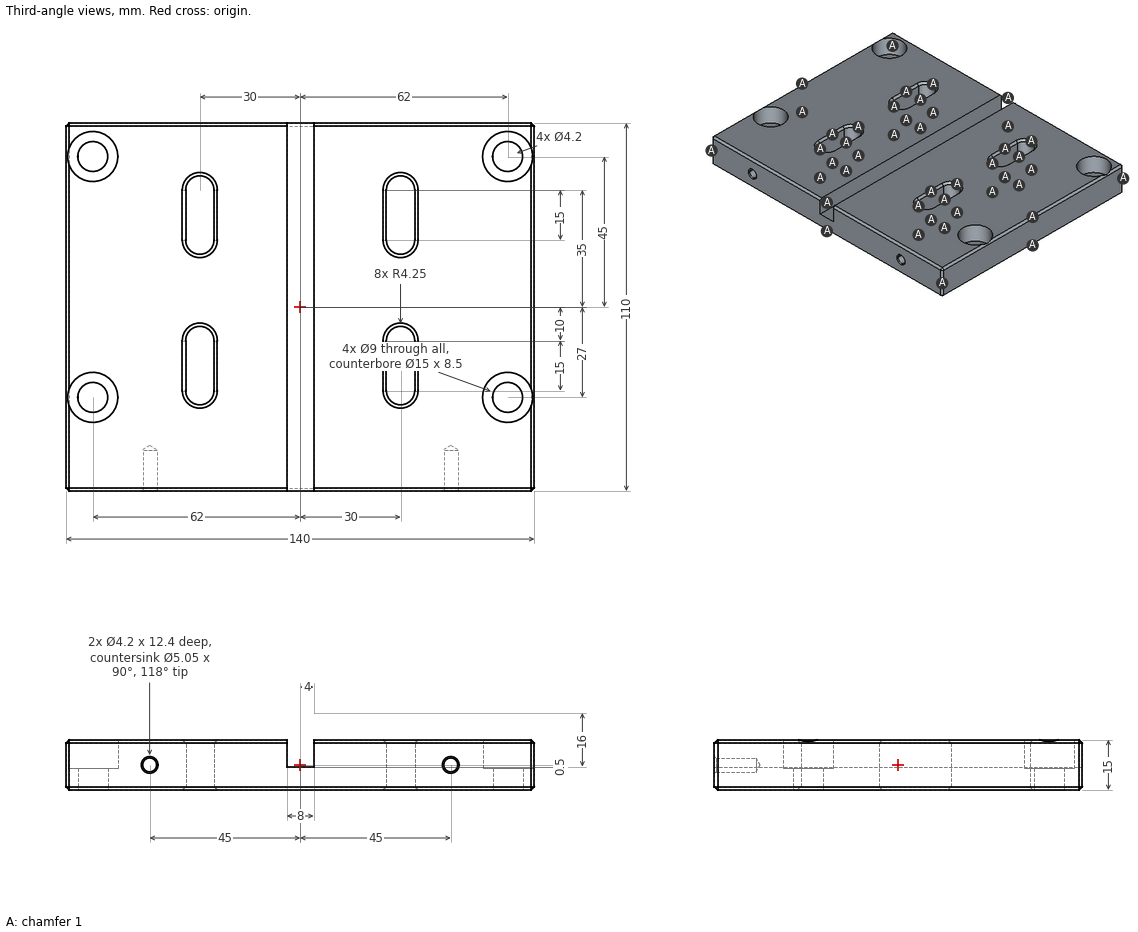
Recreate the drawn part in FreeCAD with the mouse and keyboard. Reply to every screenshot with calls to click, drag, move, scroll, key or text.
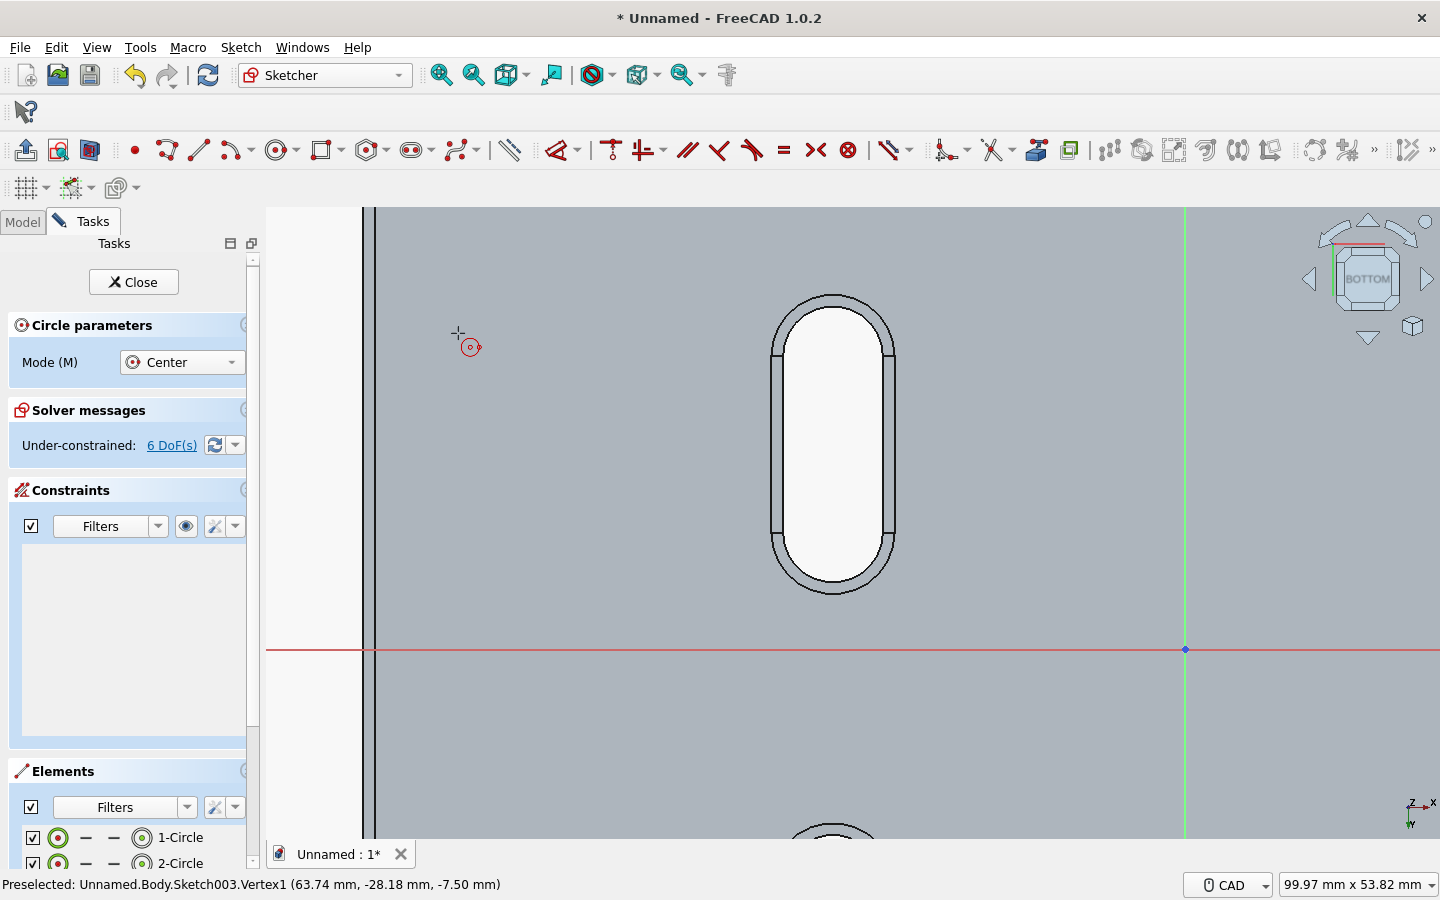
click(457, 333)
click(475, 315)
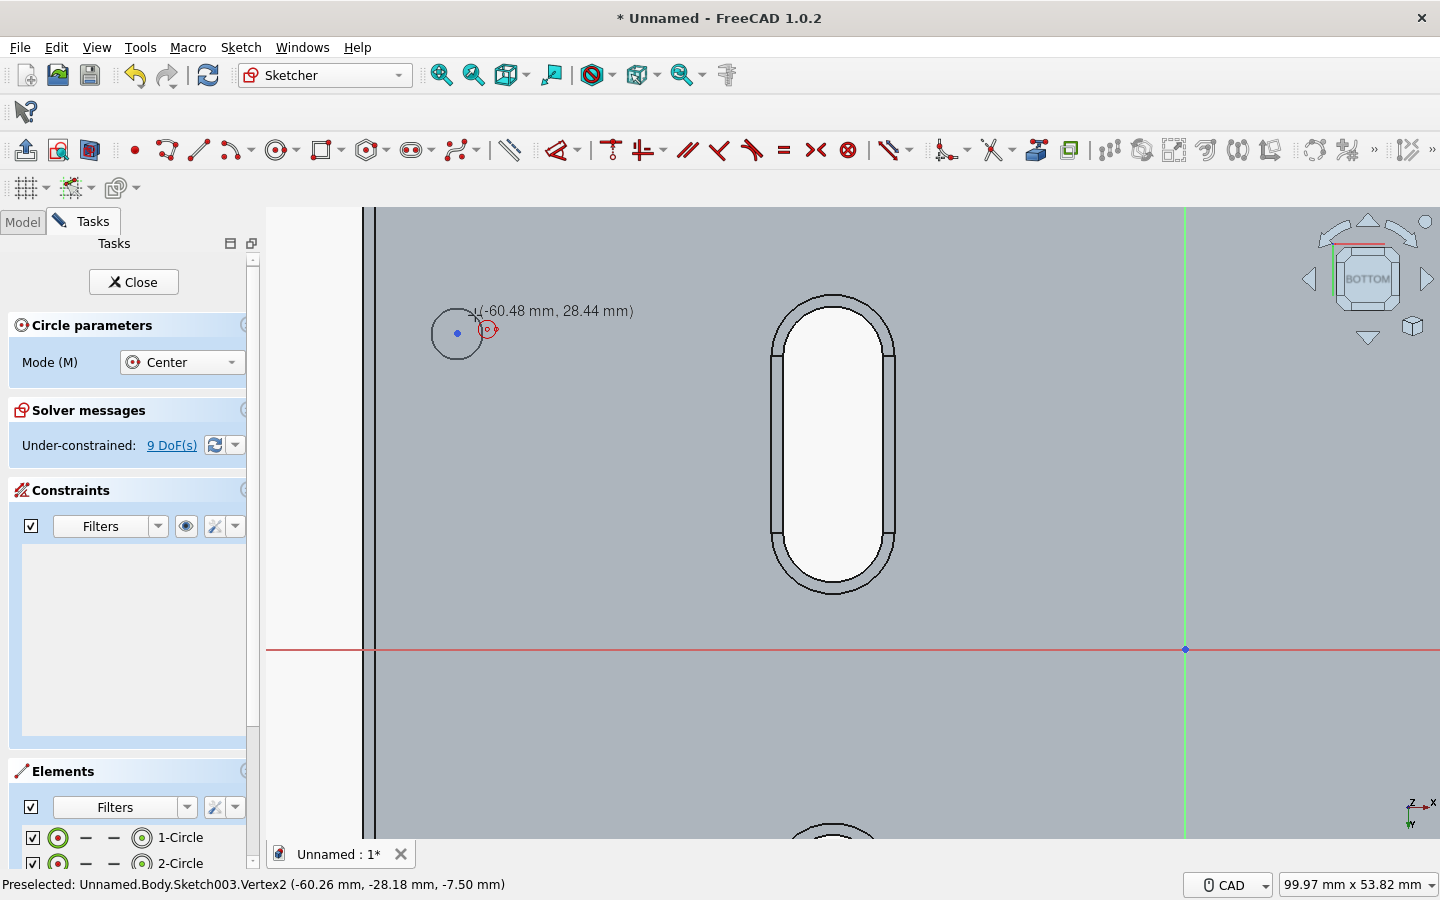
scroll(457, 333, down, 4)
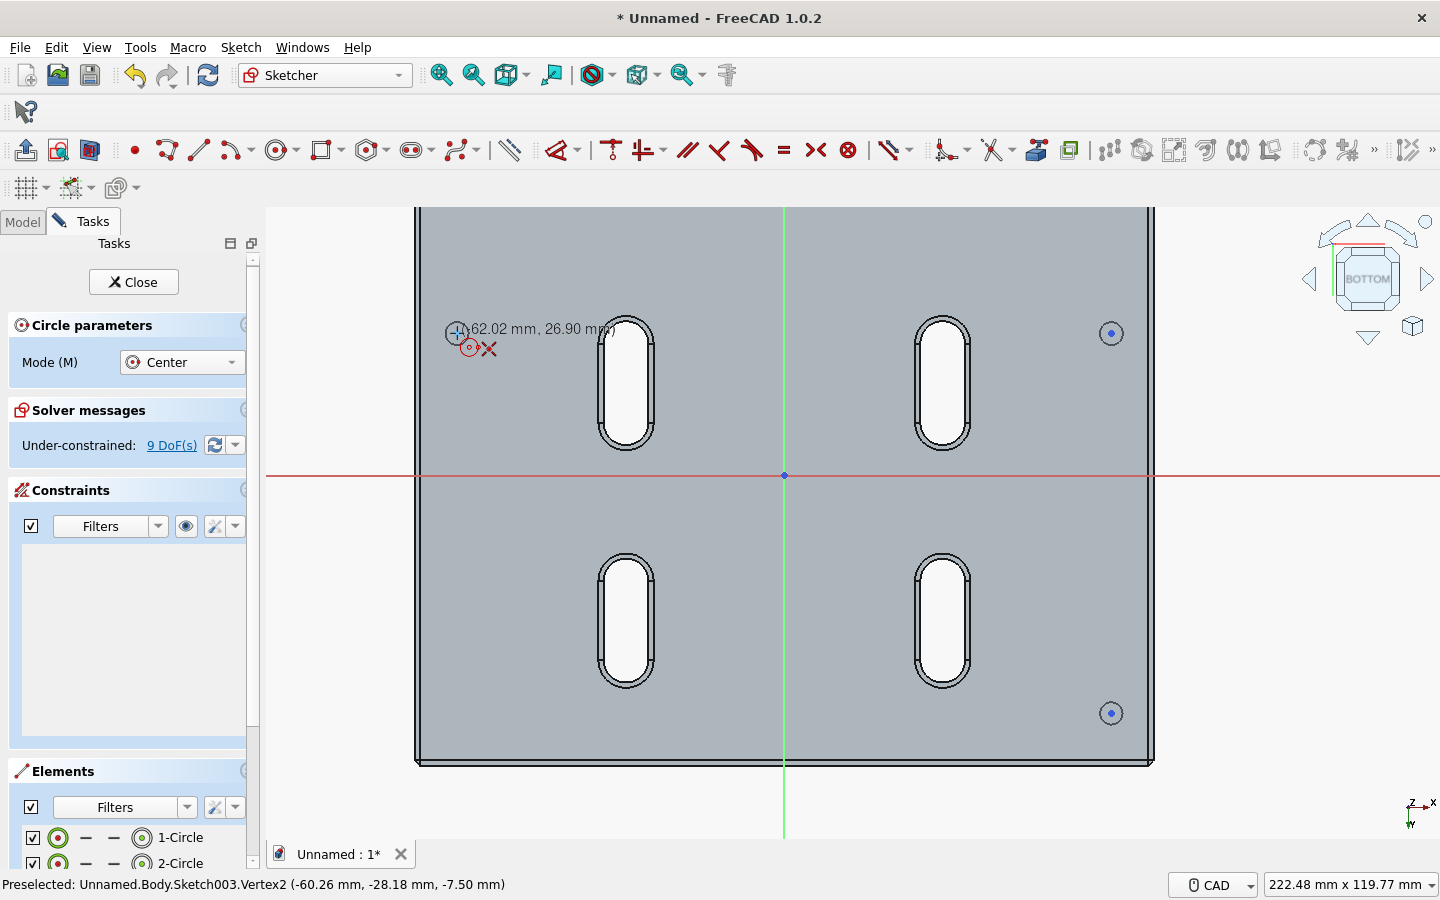
scroll(457, 713, up, 4)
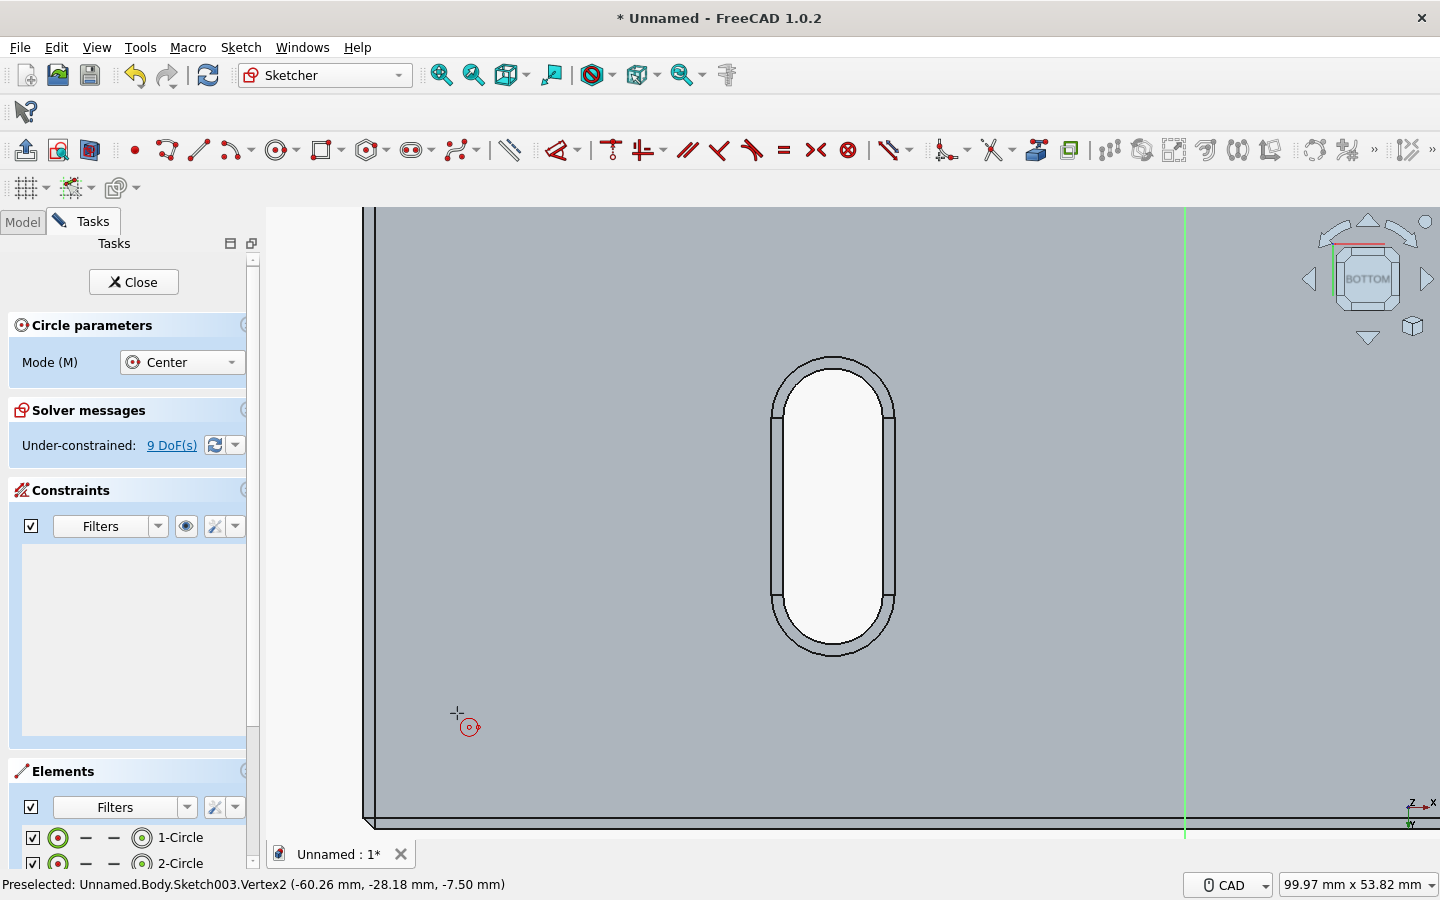
click(457, 712)
click(475, 695)
key(Escape)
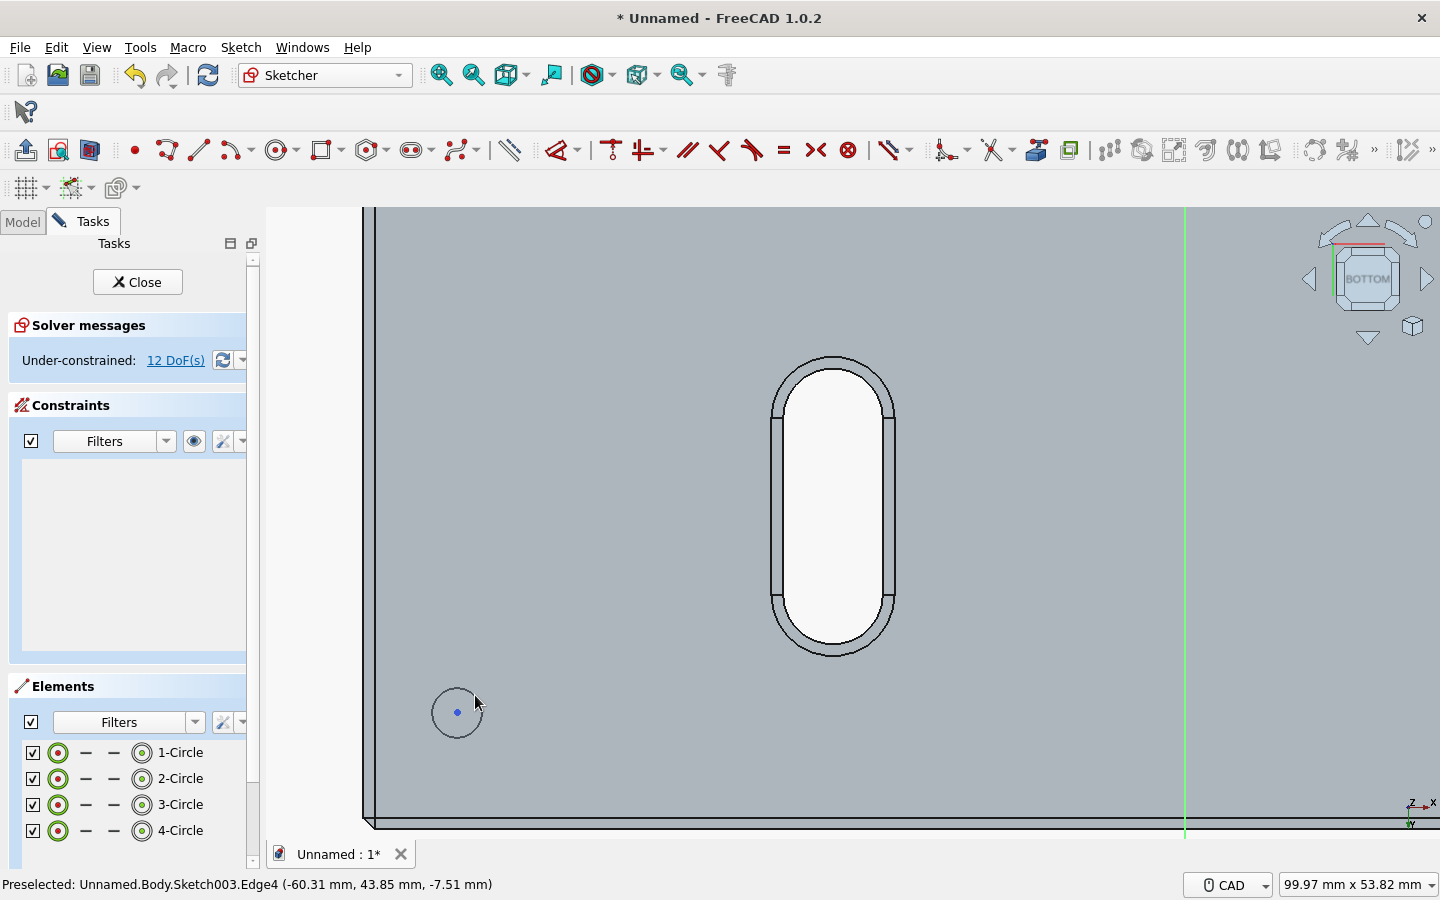
scroll(457, 714, down, 4)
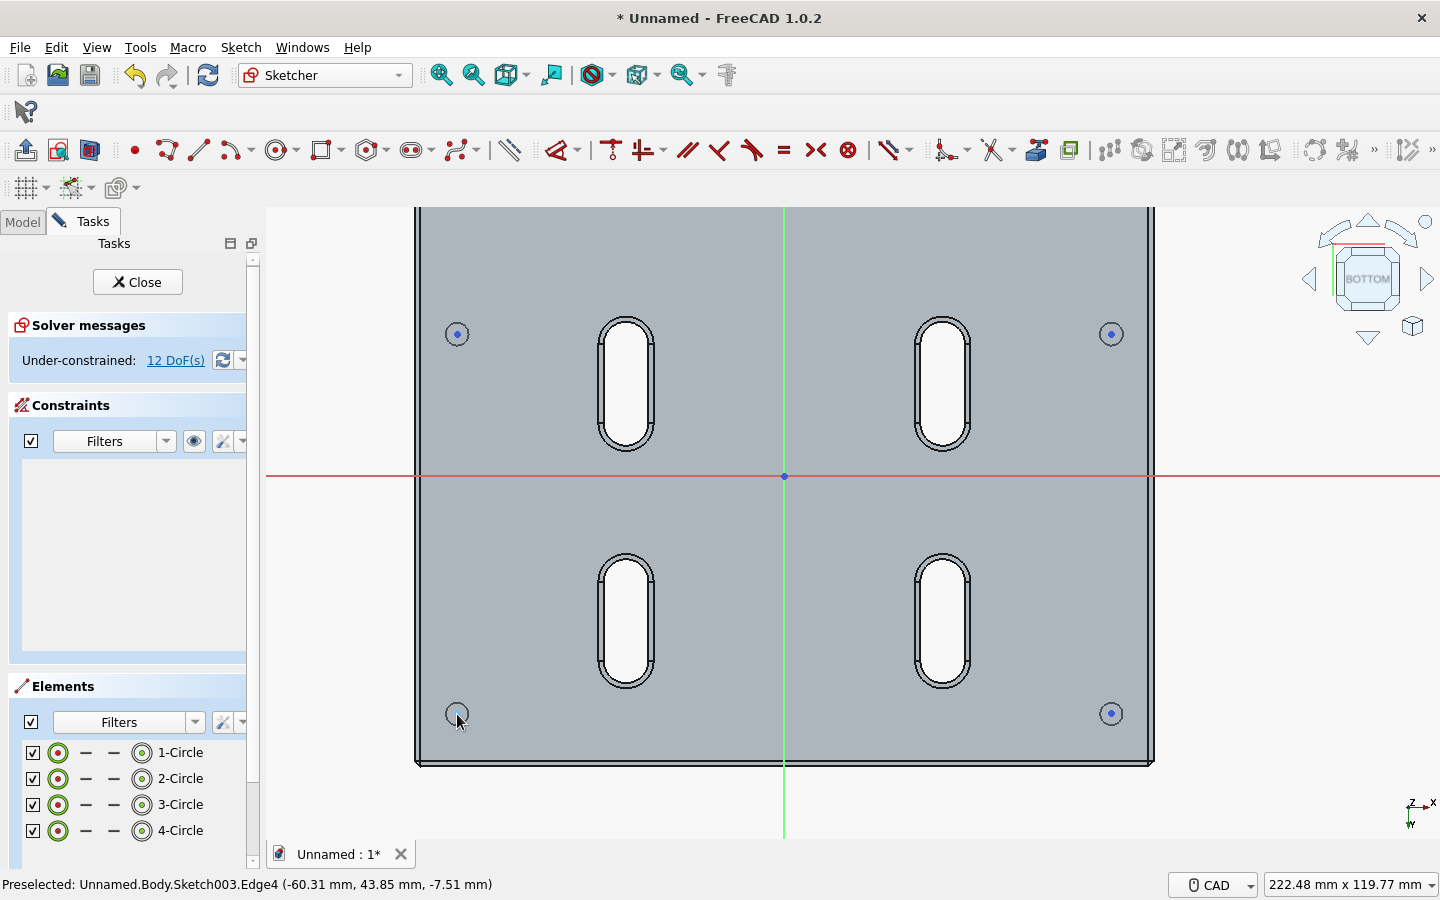
scroll(1119, 706, up, 2)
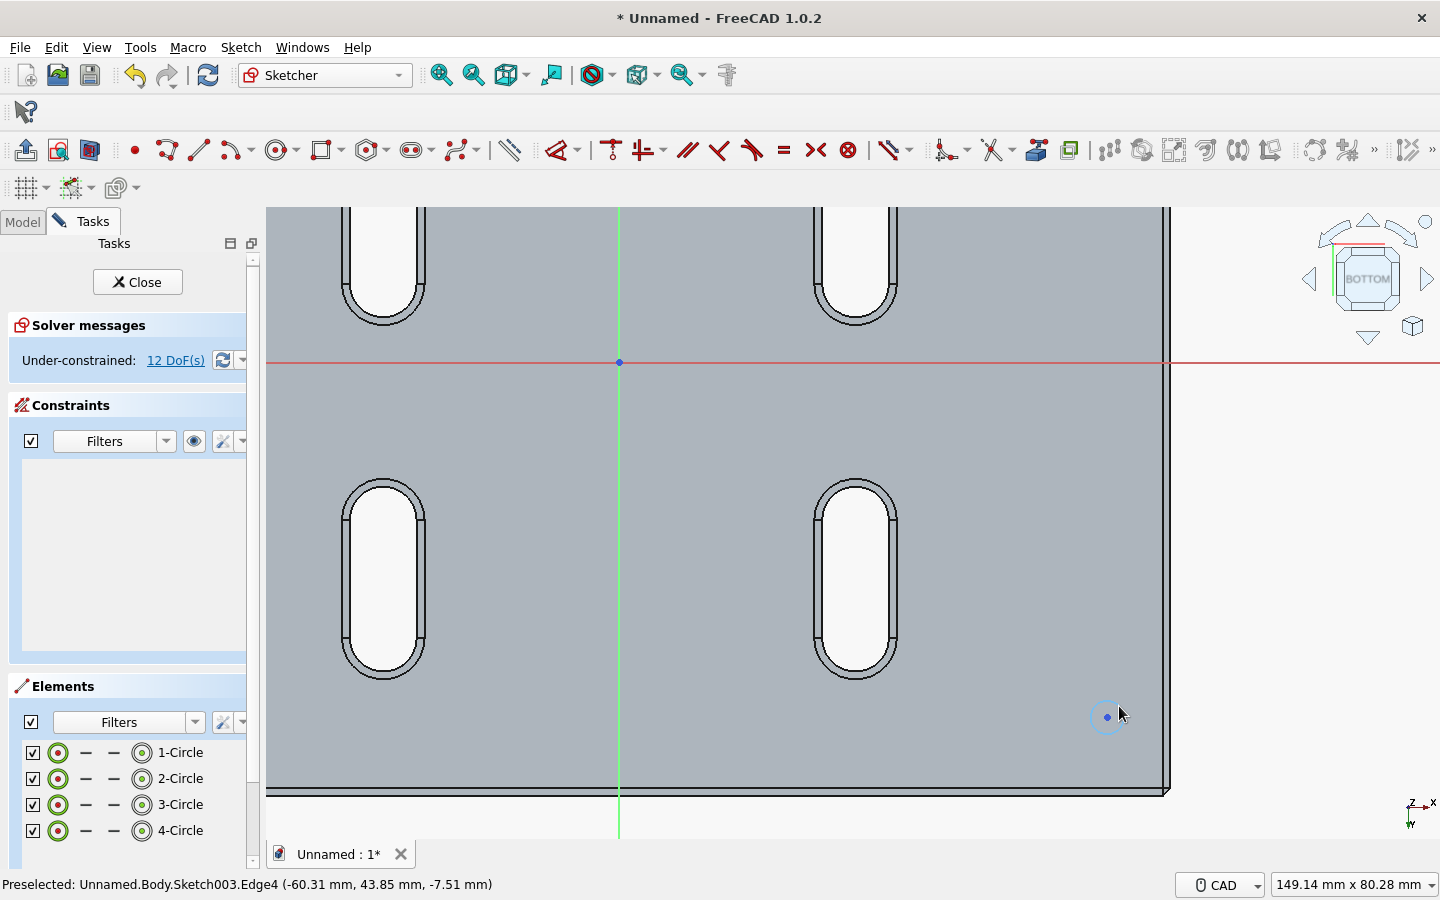
click(1119, 706)